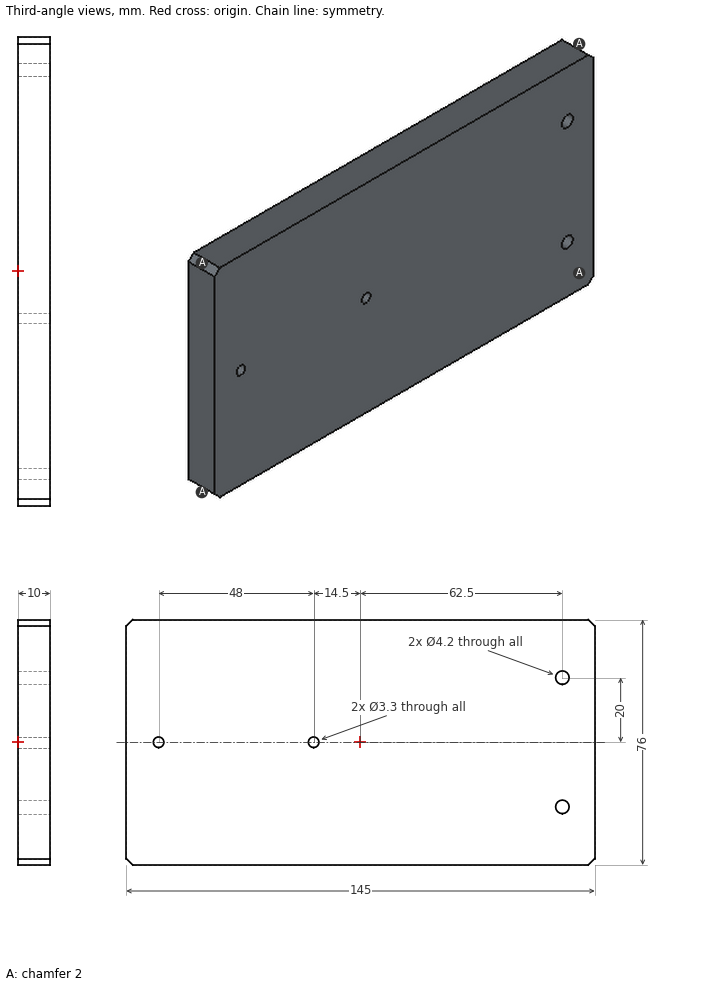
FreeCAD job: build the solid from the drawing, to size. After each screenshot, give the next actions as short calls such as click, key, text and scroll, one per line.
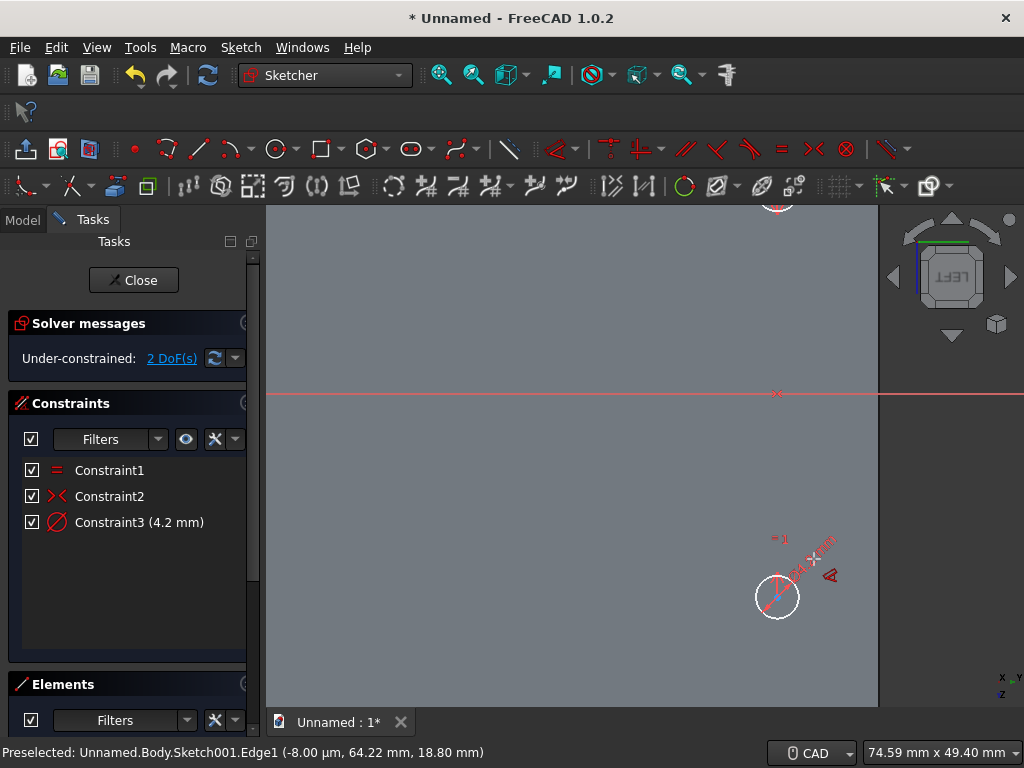
click(777, 597)
click(811, 495)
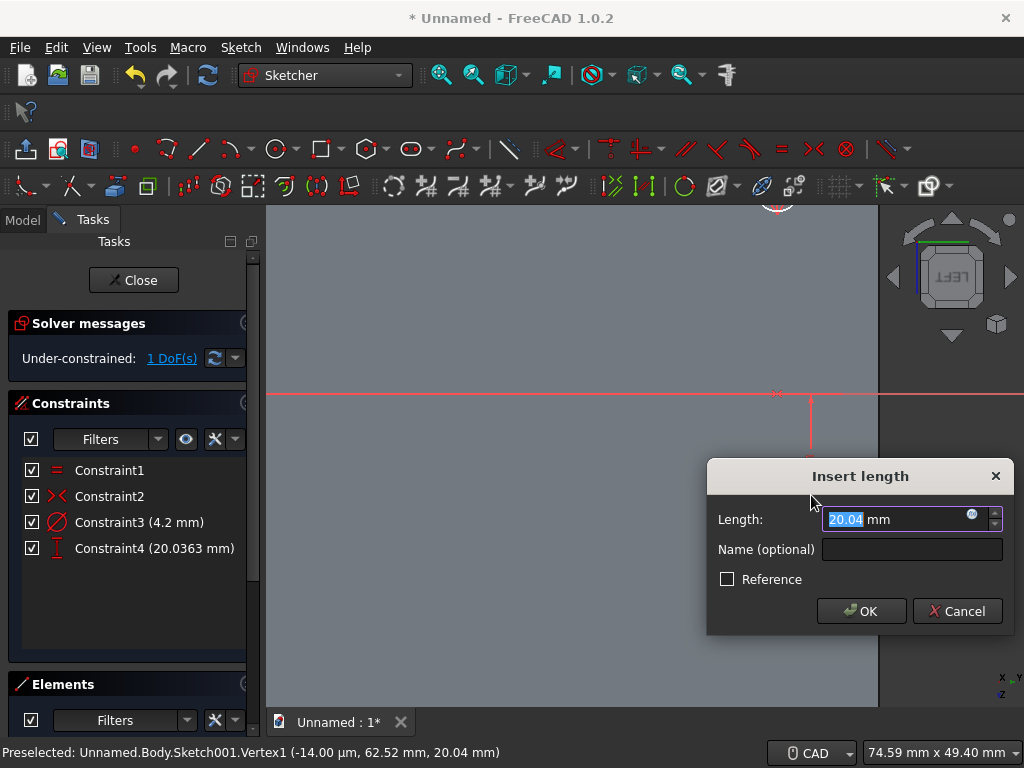
text(20)
key(Return)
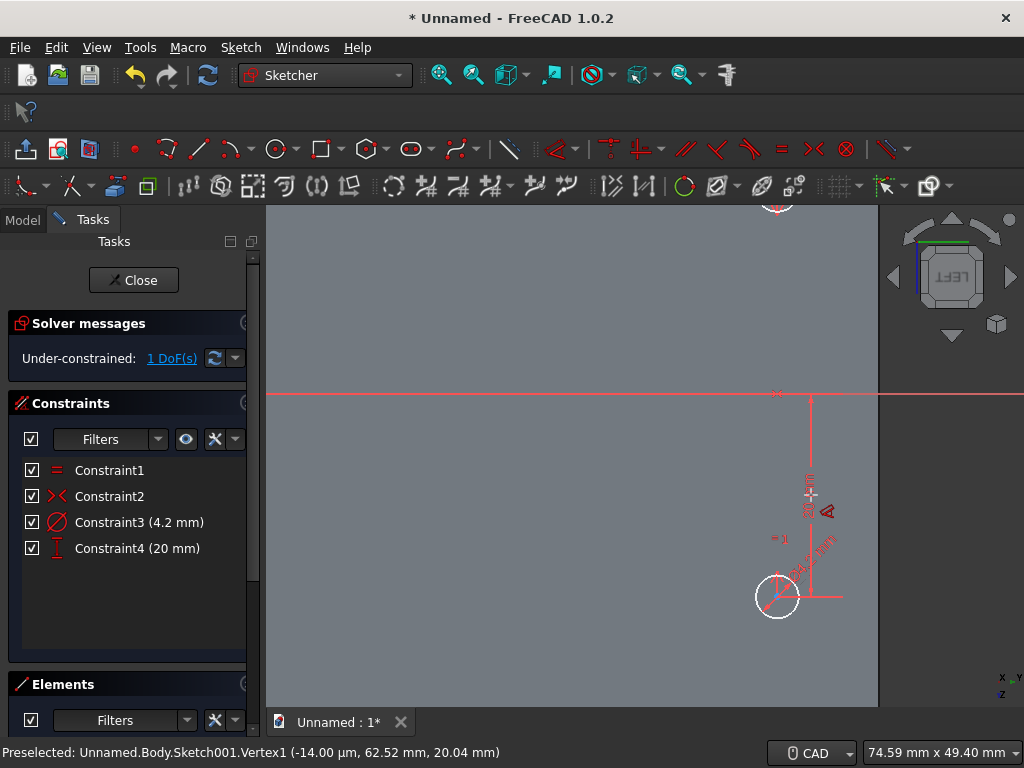
click(777, 597)
click(536, 631)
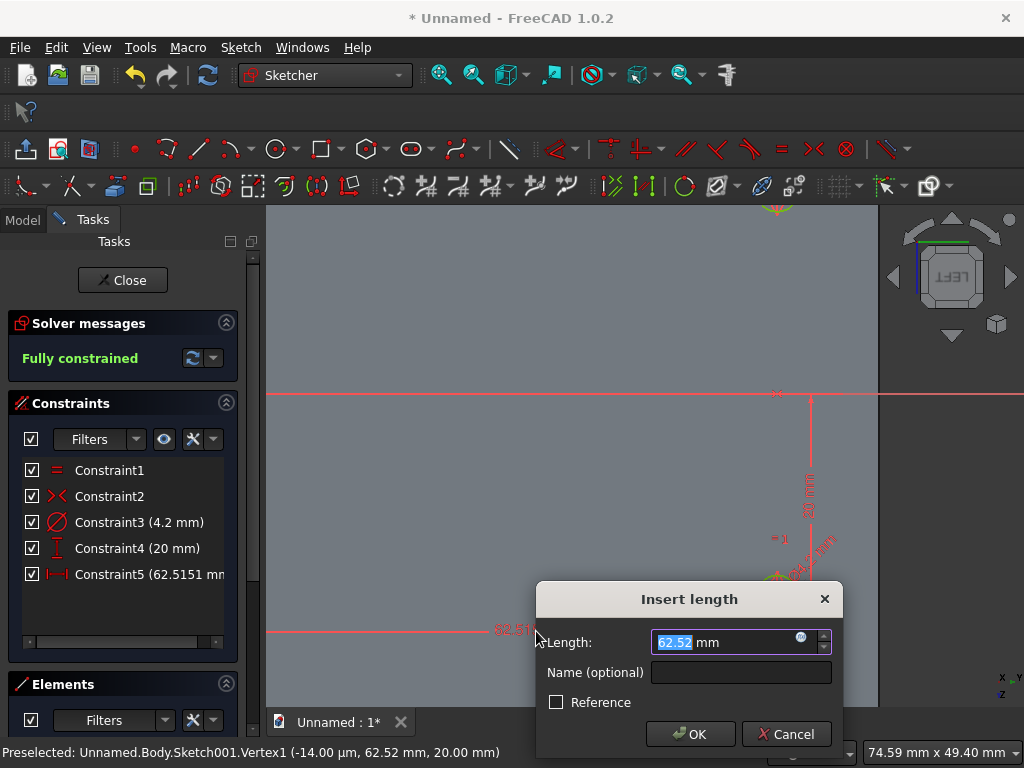
text(62.5)
key(Return)
key(Escape)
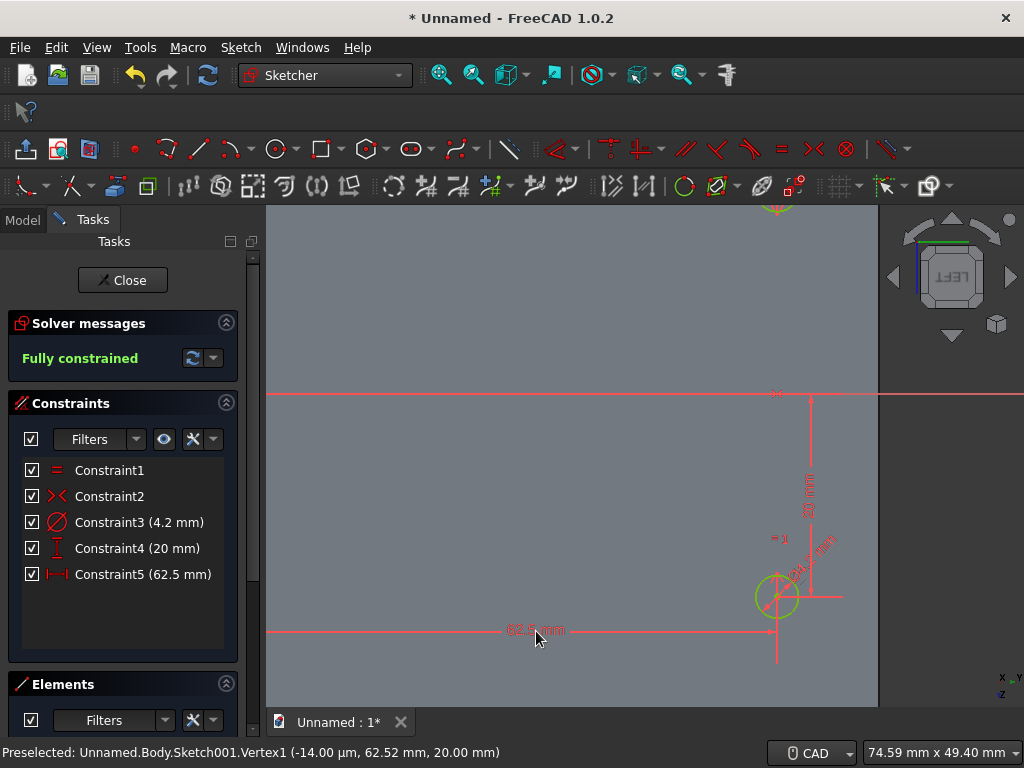
click(123, 280)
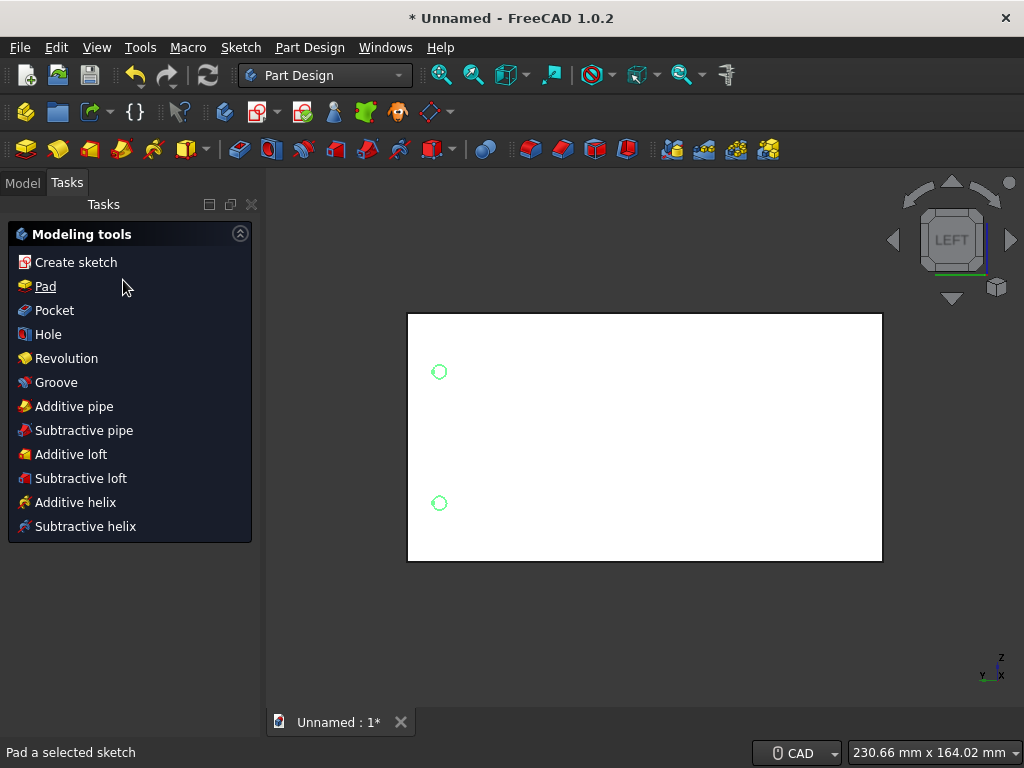
click(272, 150)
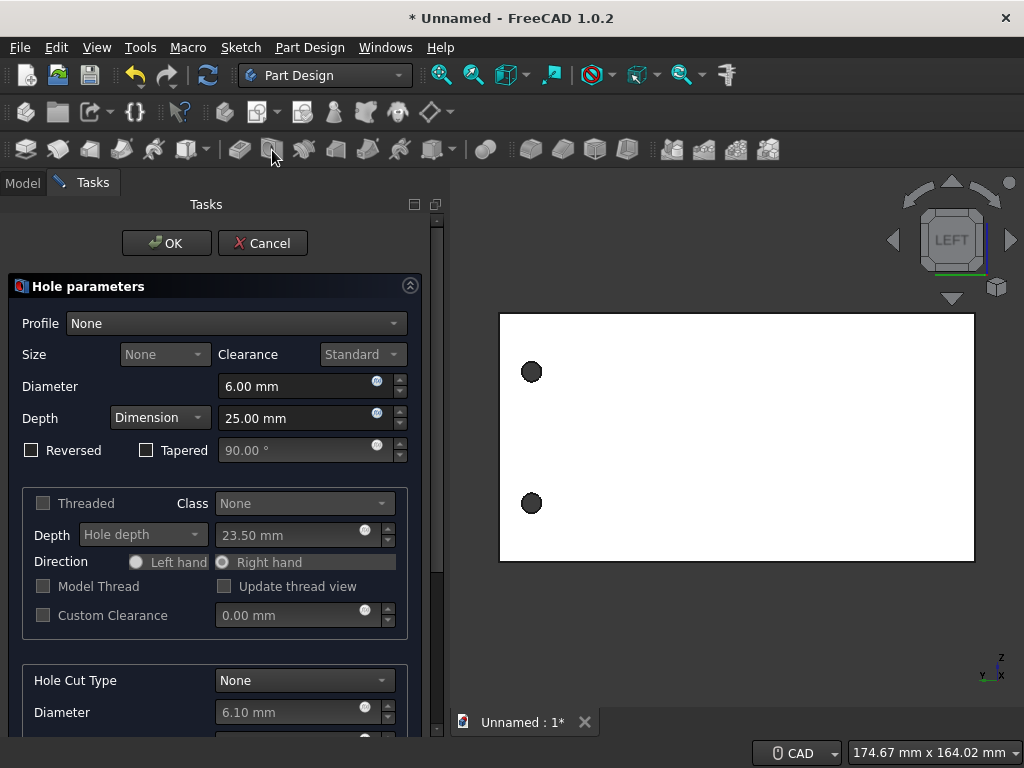
triple_click(305, 386)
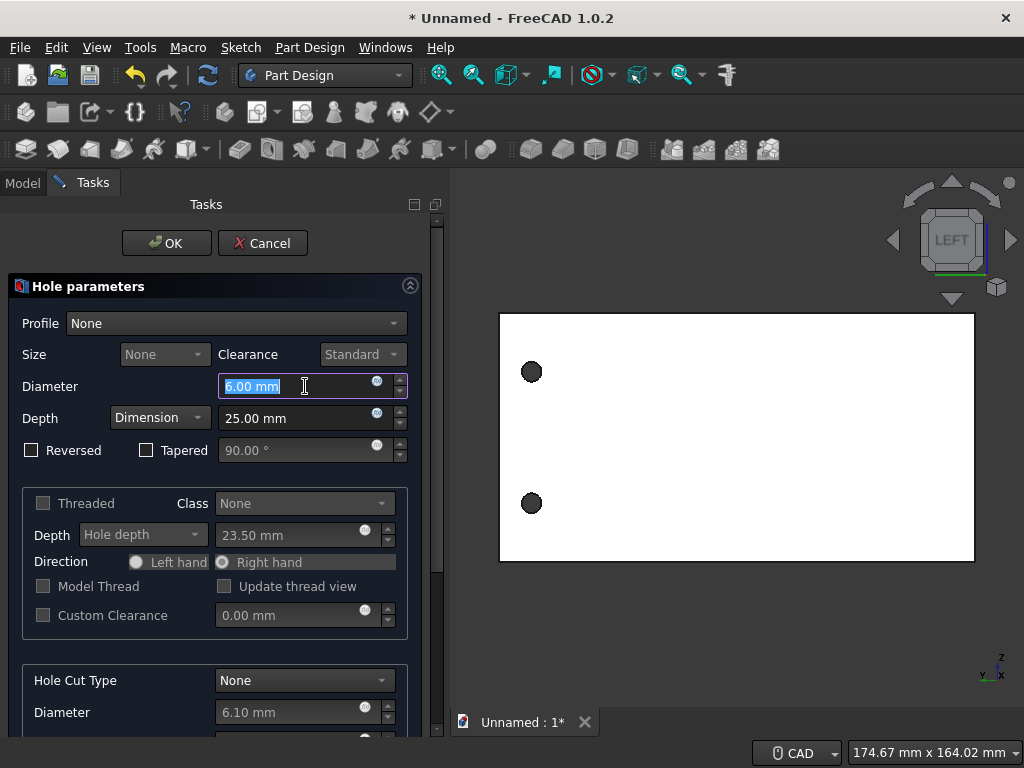
text(4.2)
key(Tab)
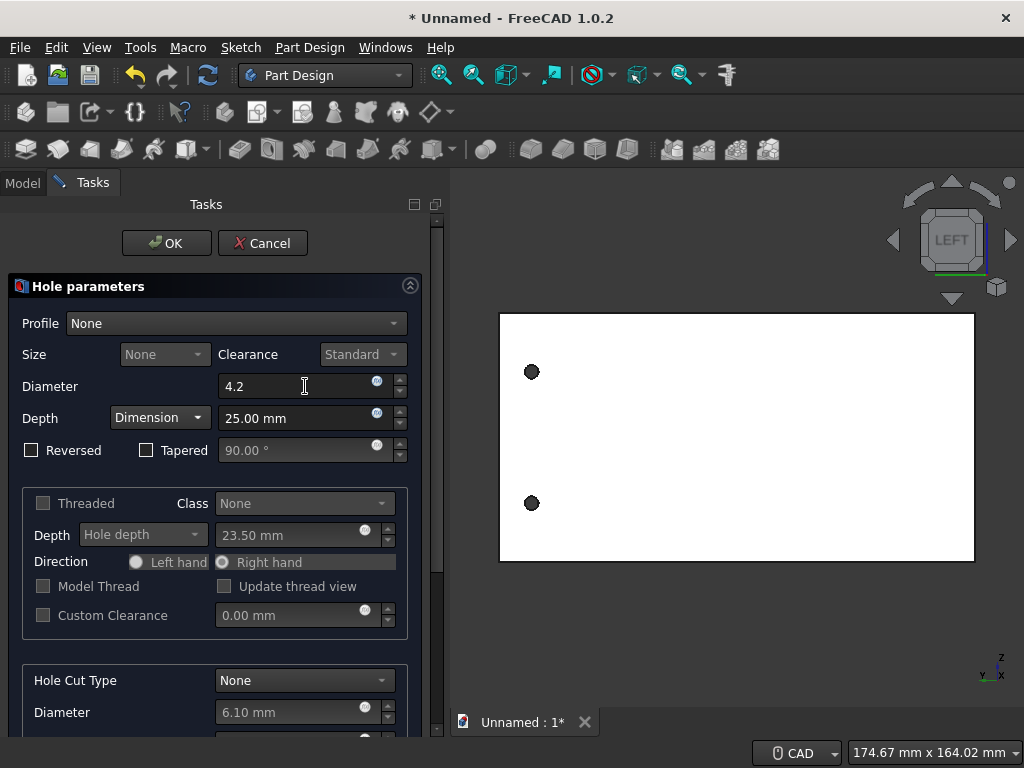
click(161, 418)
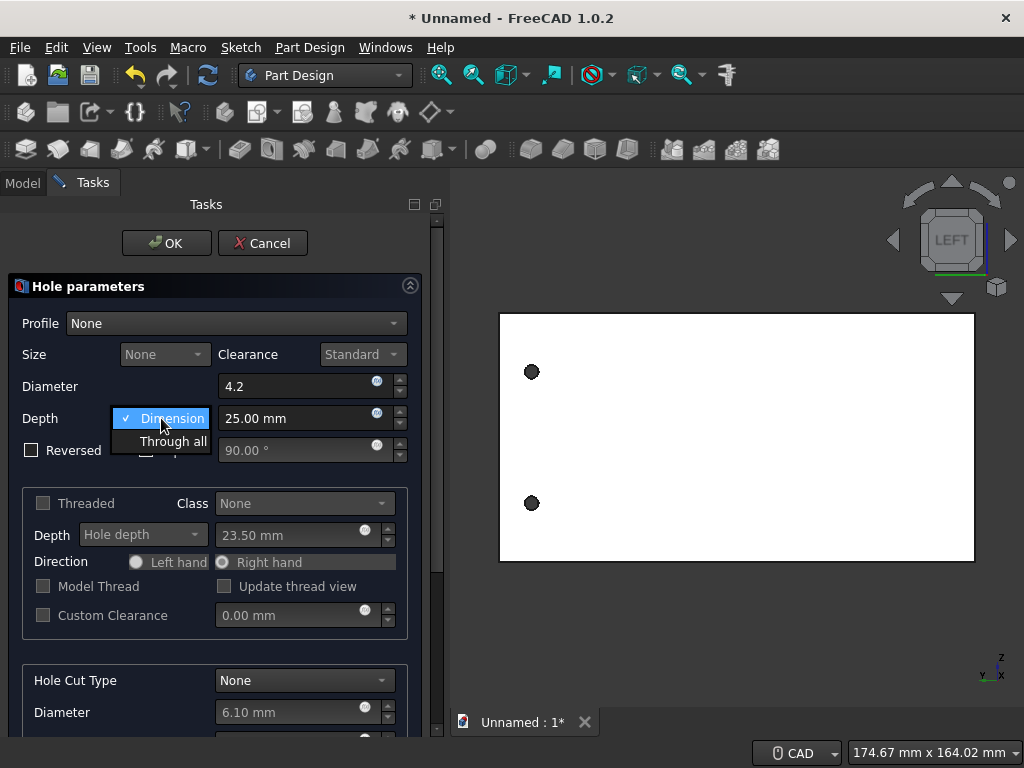
click(160, 442)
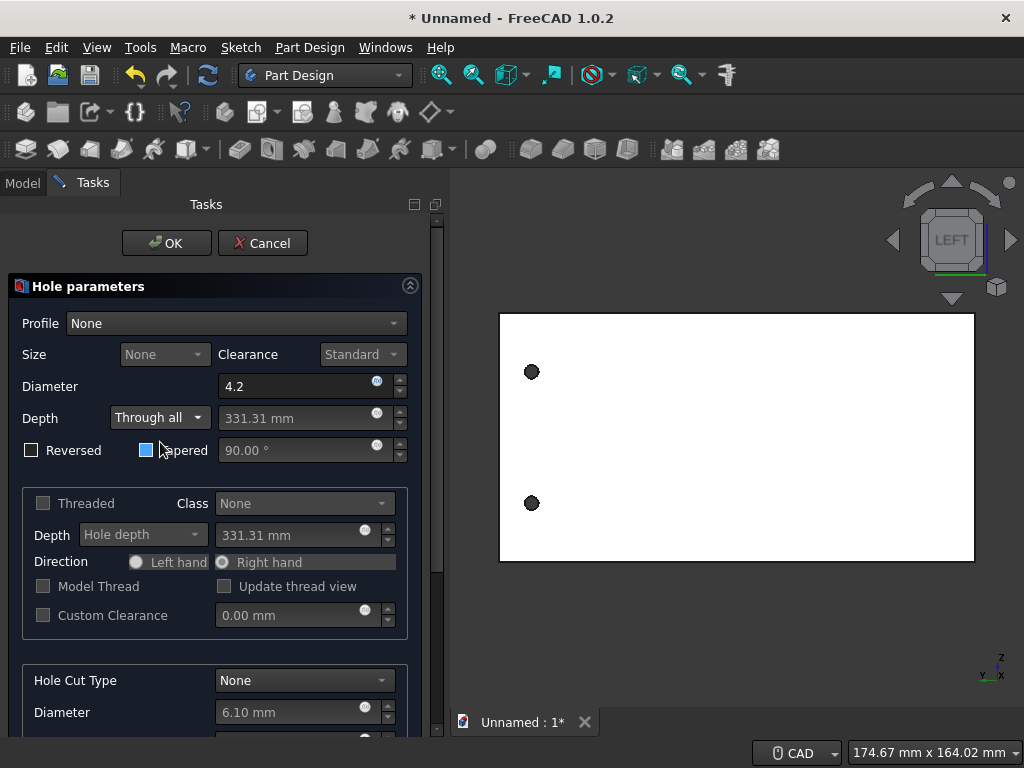
click(167, 243)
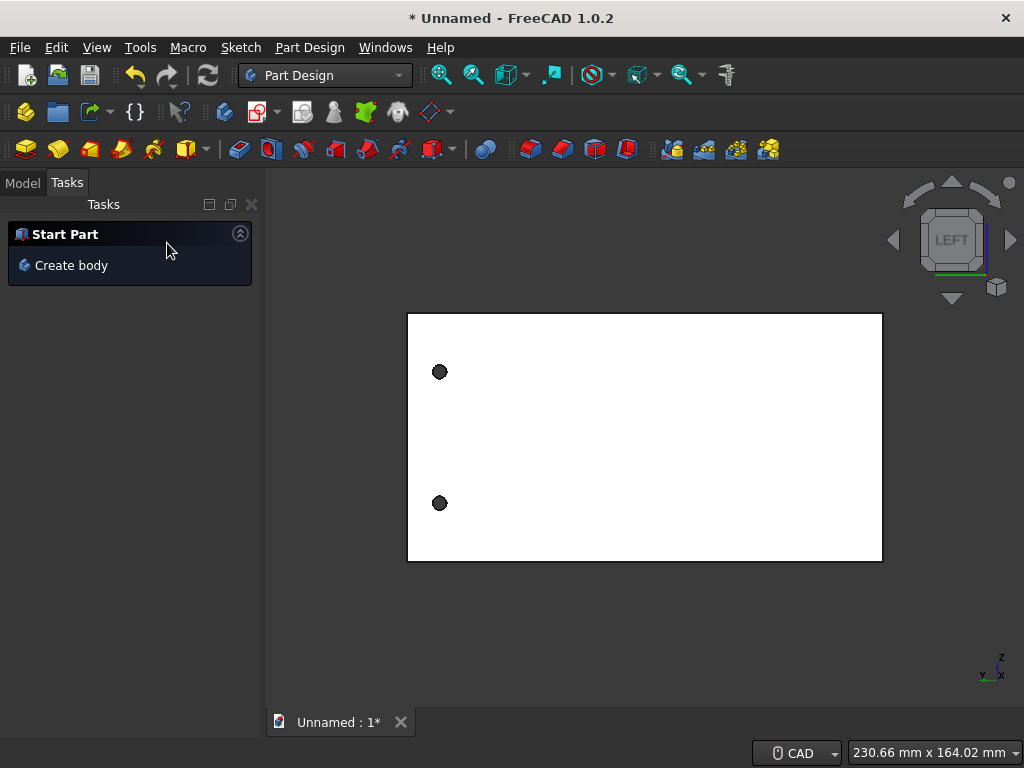
click(258, 112)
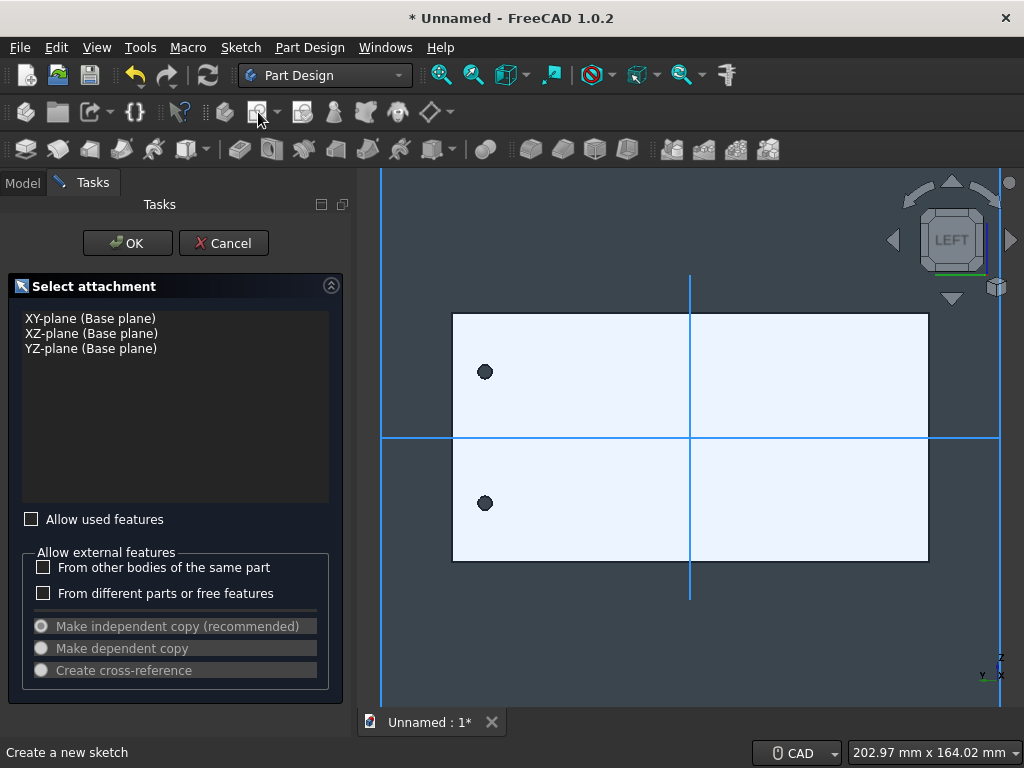
click(82, 348)